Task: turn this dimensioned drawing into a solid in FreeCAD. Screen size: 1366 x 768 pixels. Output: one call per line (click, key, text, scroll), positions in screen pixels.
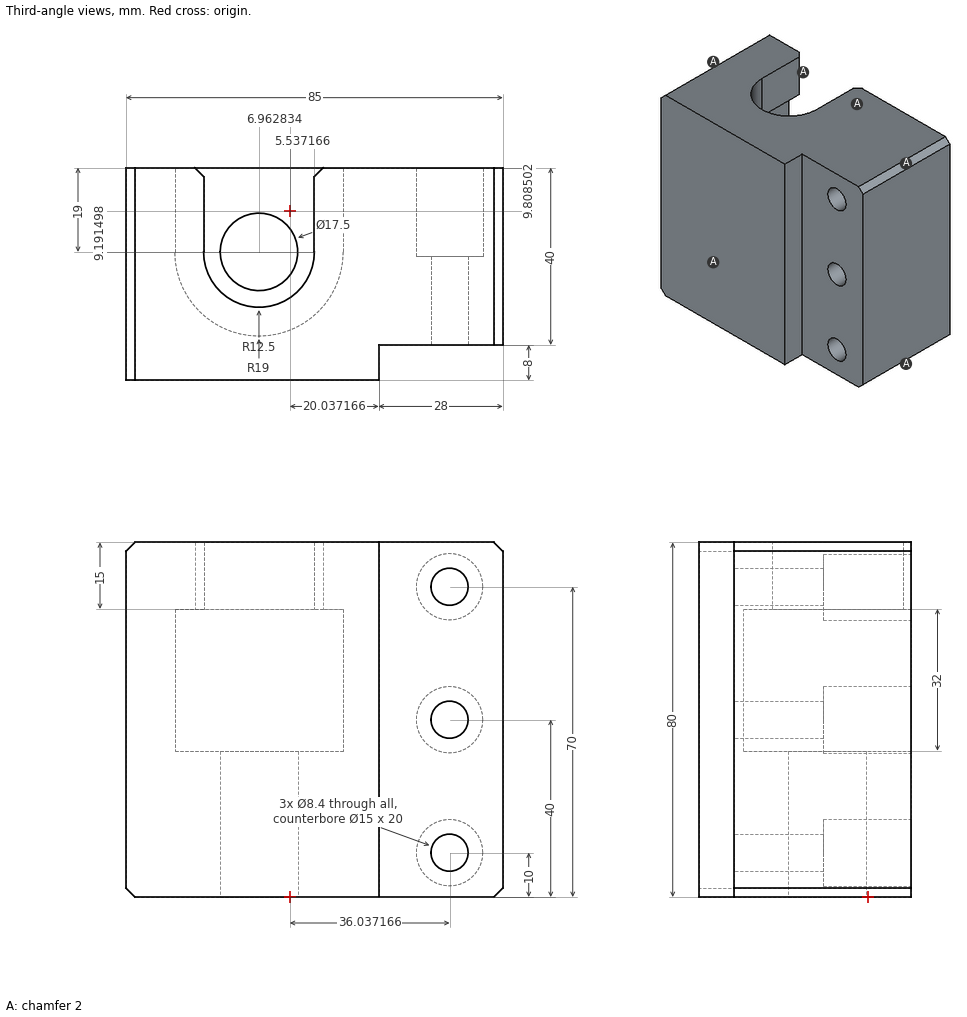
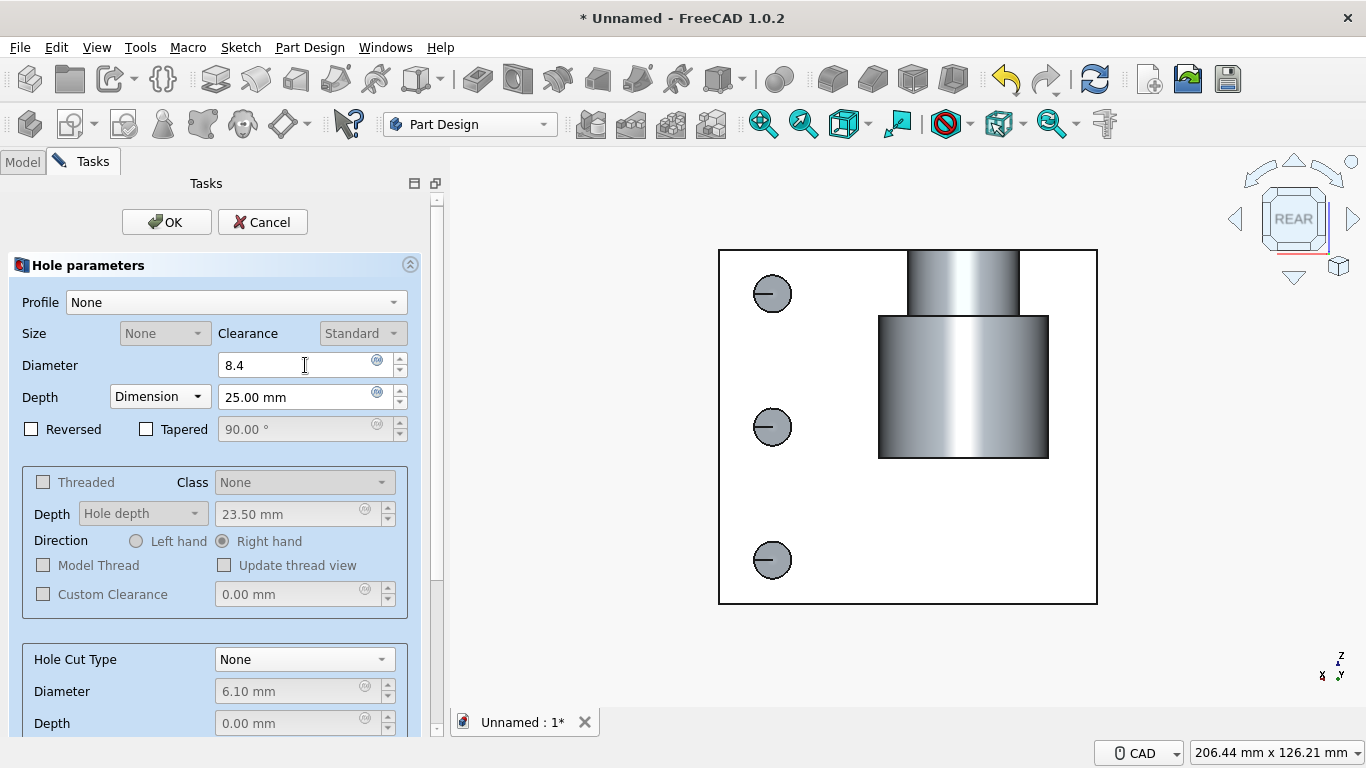
click(161, 396)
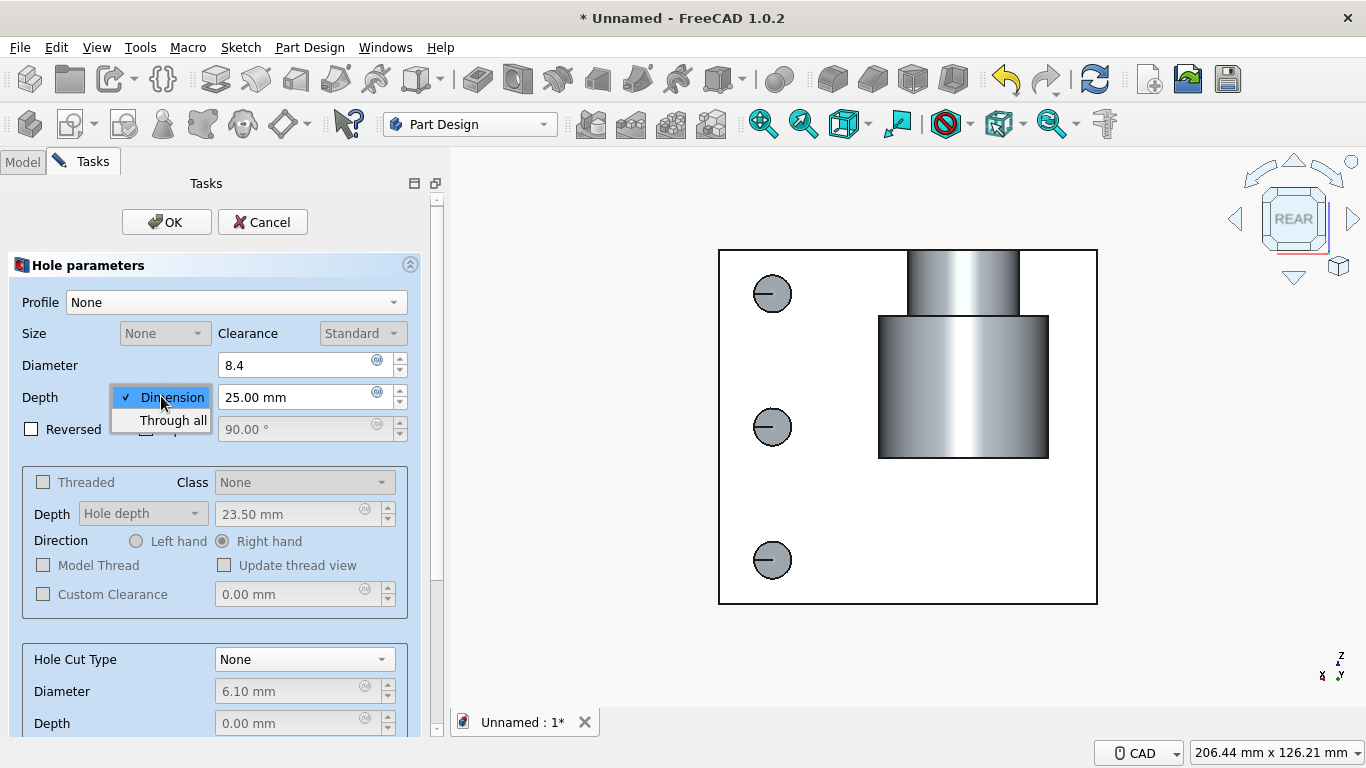
click(160, 420)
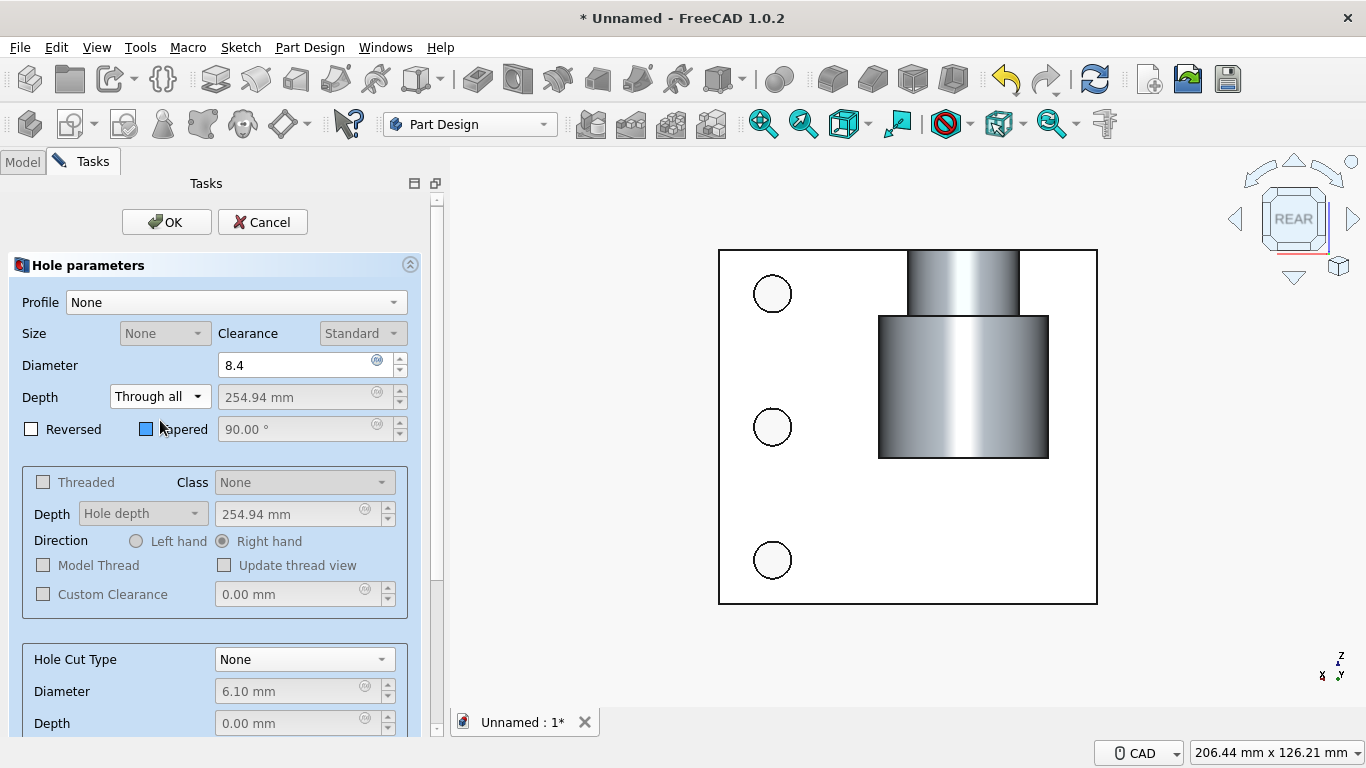
click(306, 660)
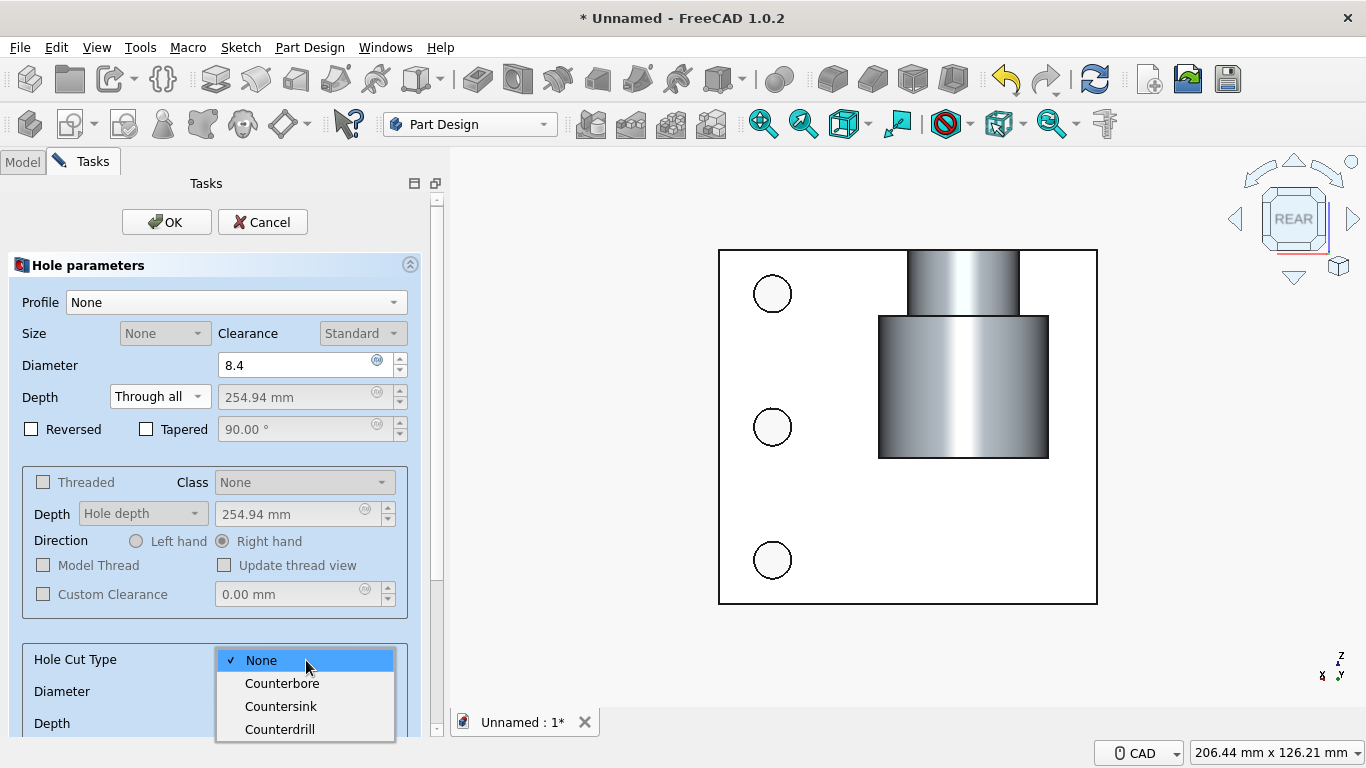
click(304, 684)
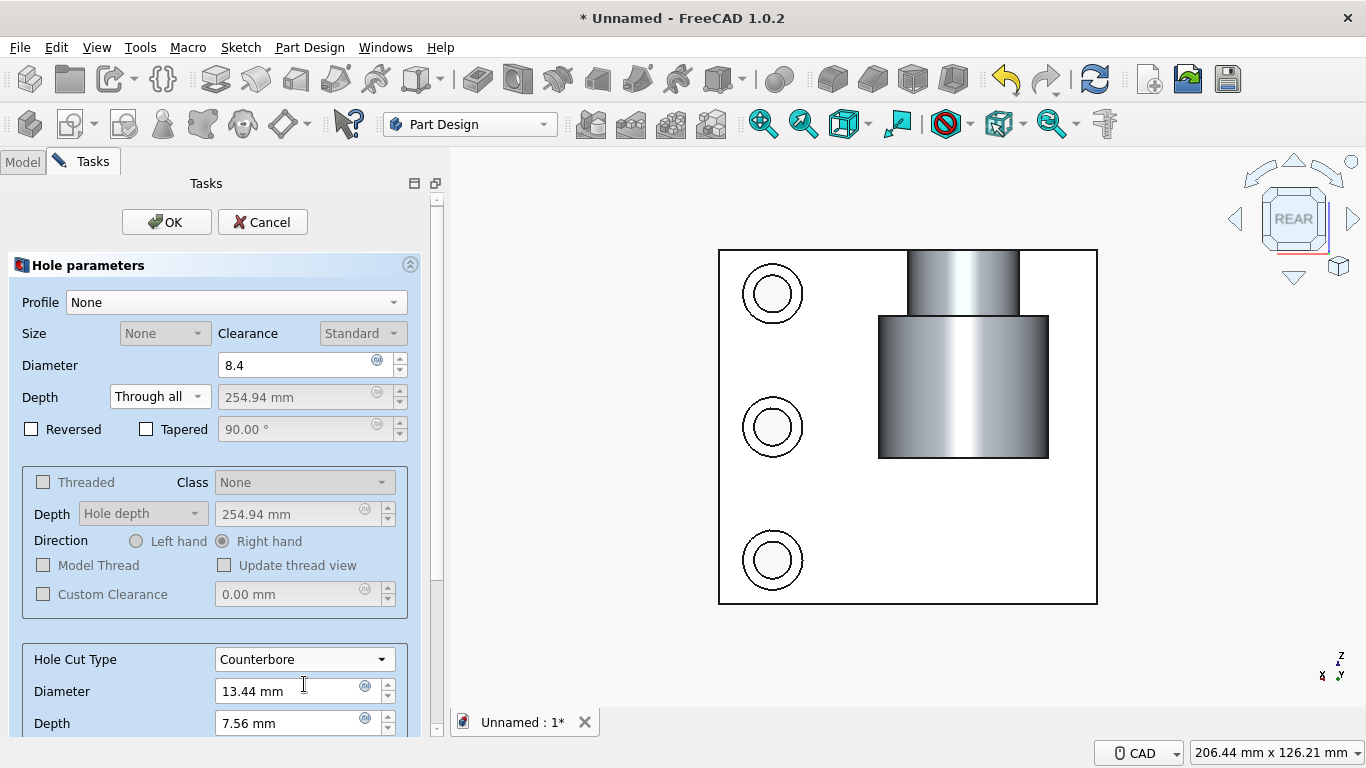
triple_click(298, 691)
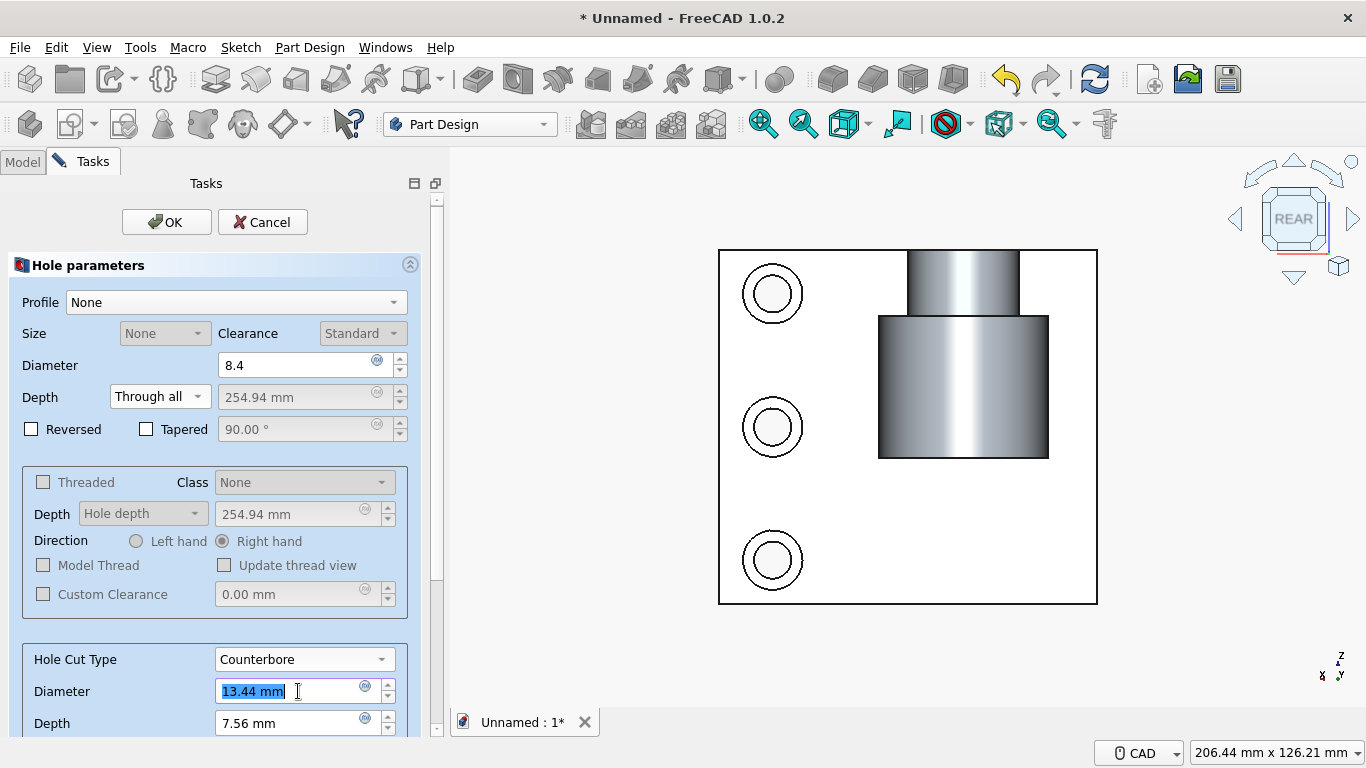
text(15)
key(Tab)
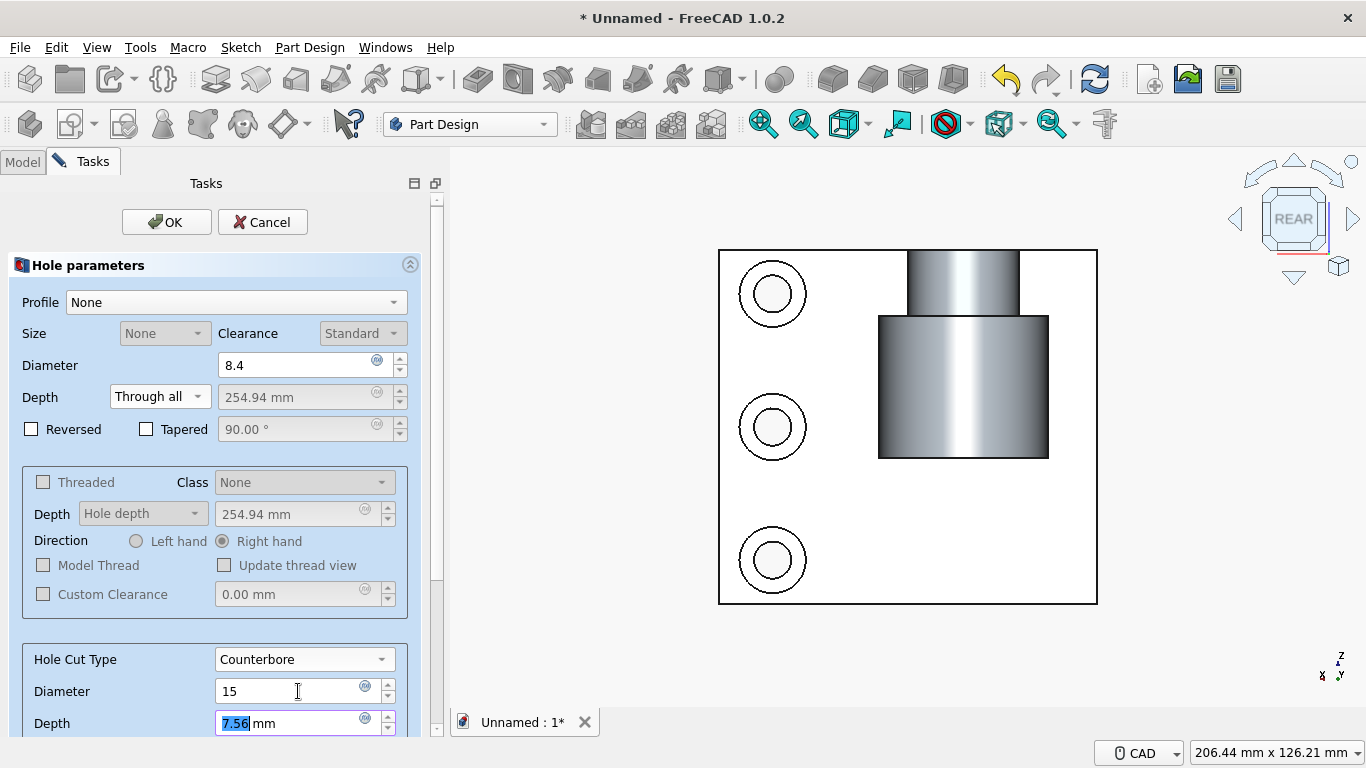
text(20)
key(Tab)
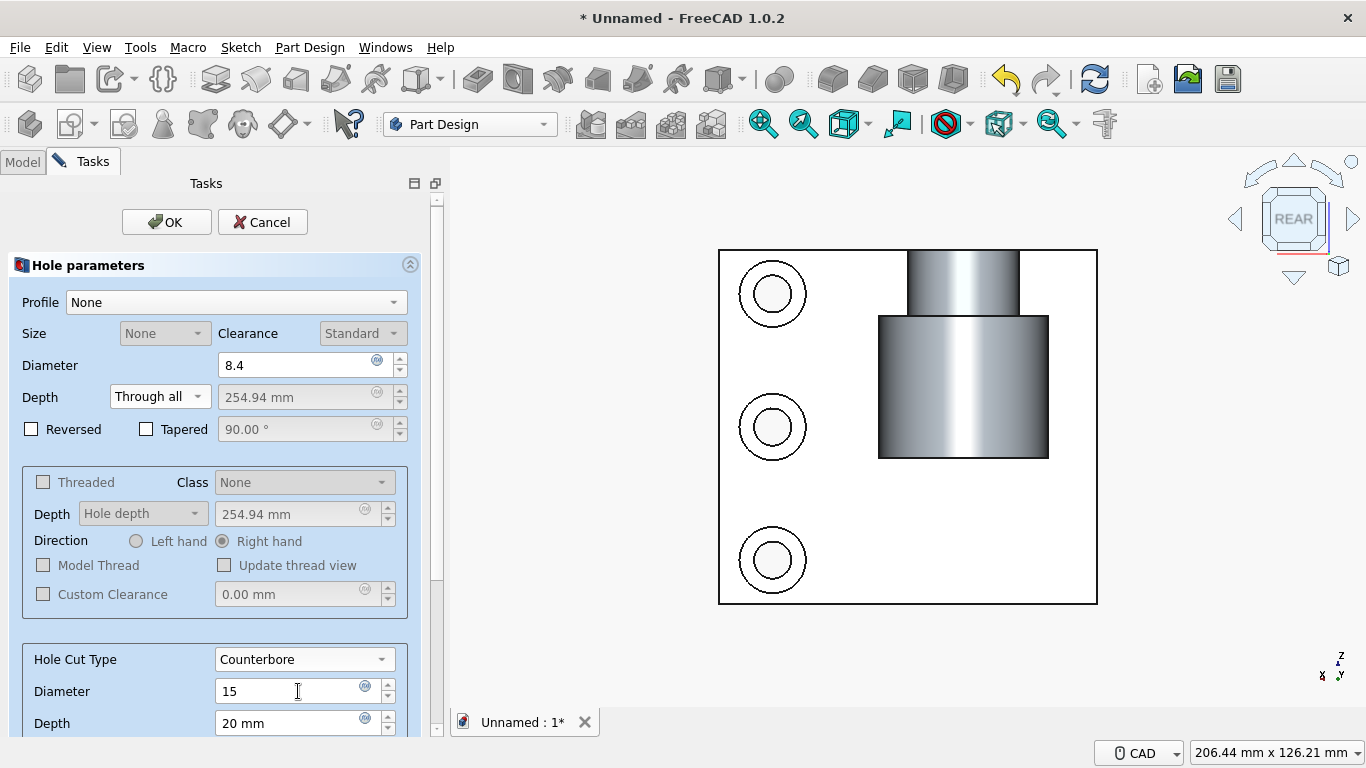
click(167, 222)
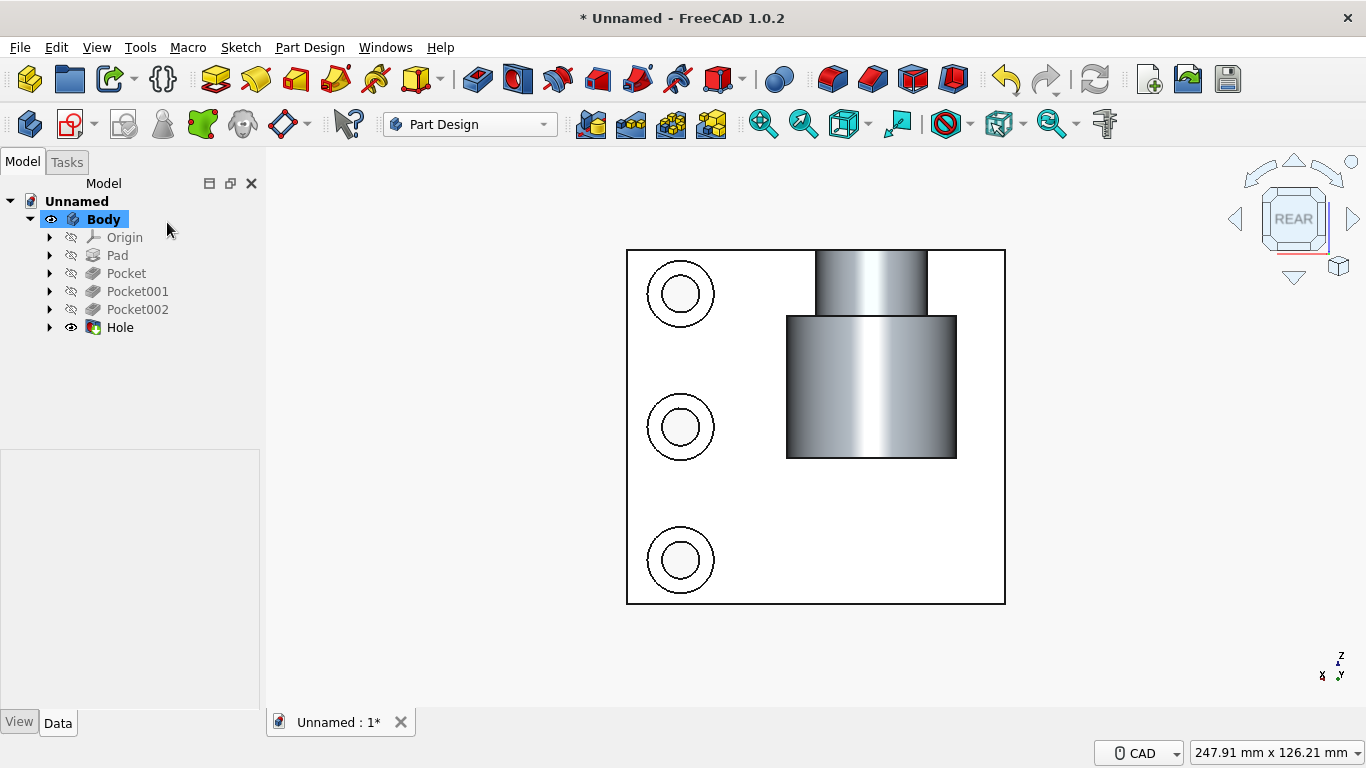
click(816, 282)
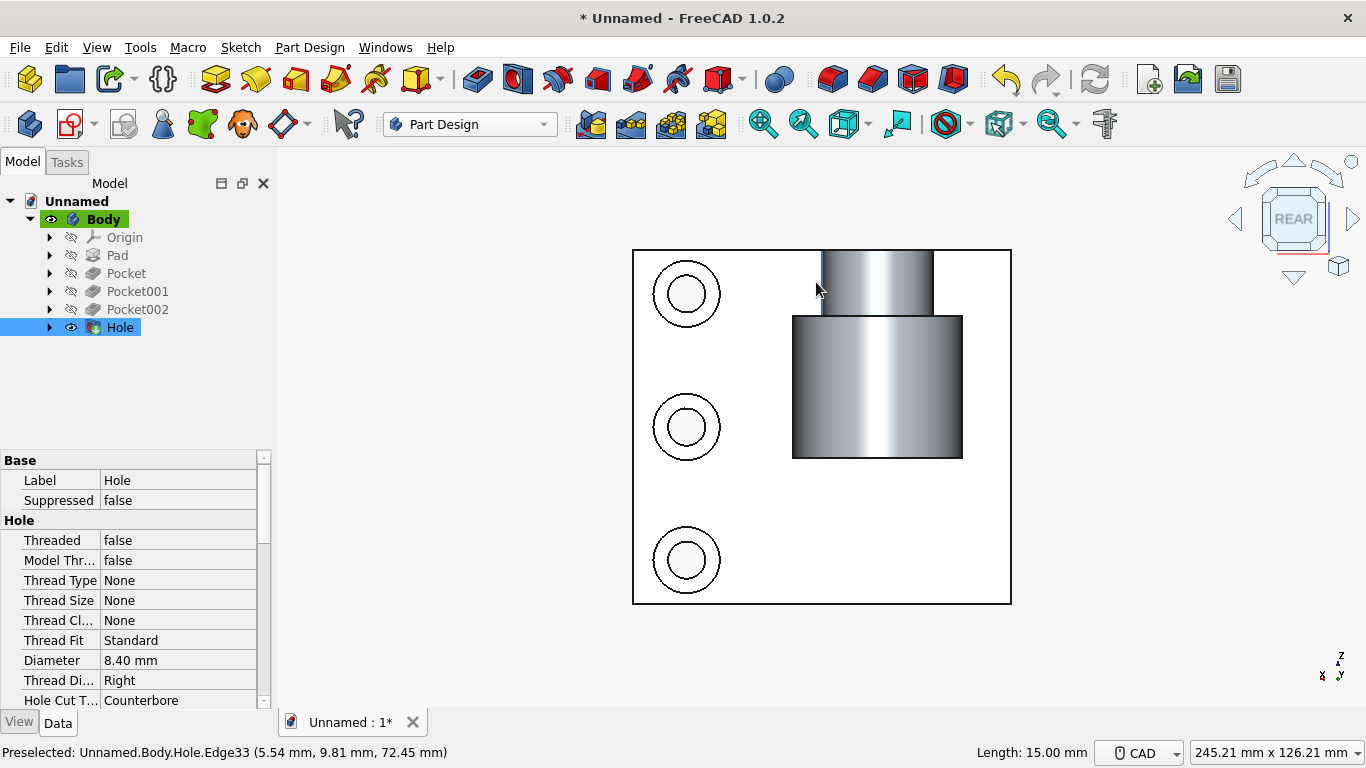
key(0)